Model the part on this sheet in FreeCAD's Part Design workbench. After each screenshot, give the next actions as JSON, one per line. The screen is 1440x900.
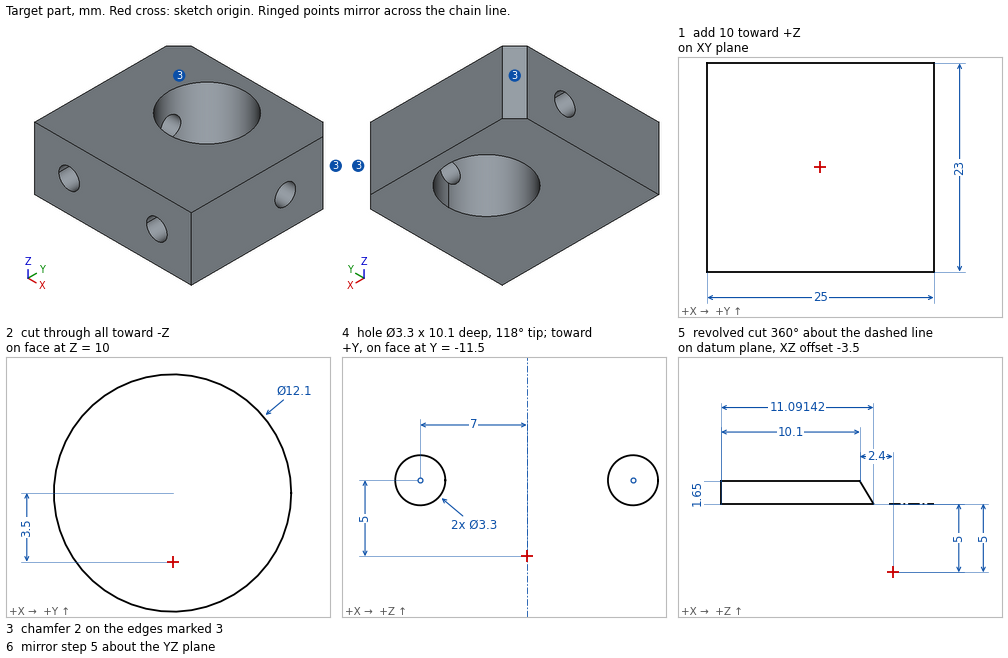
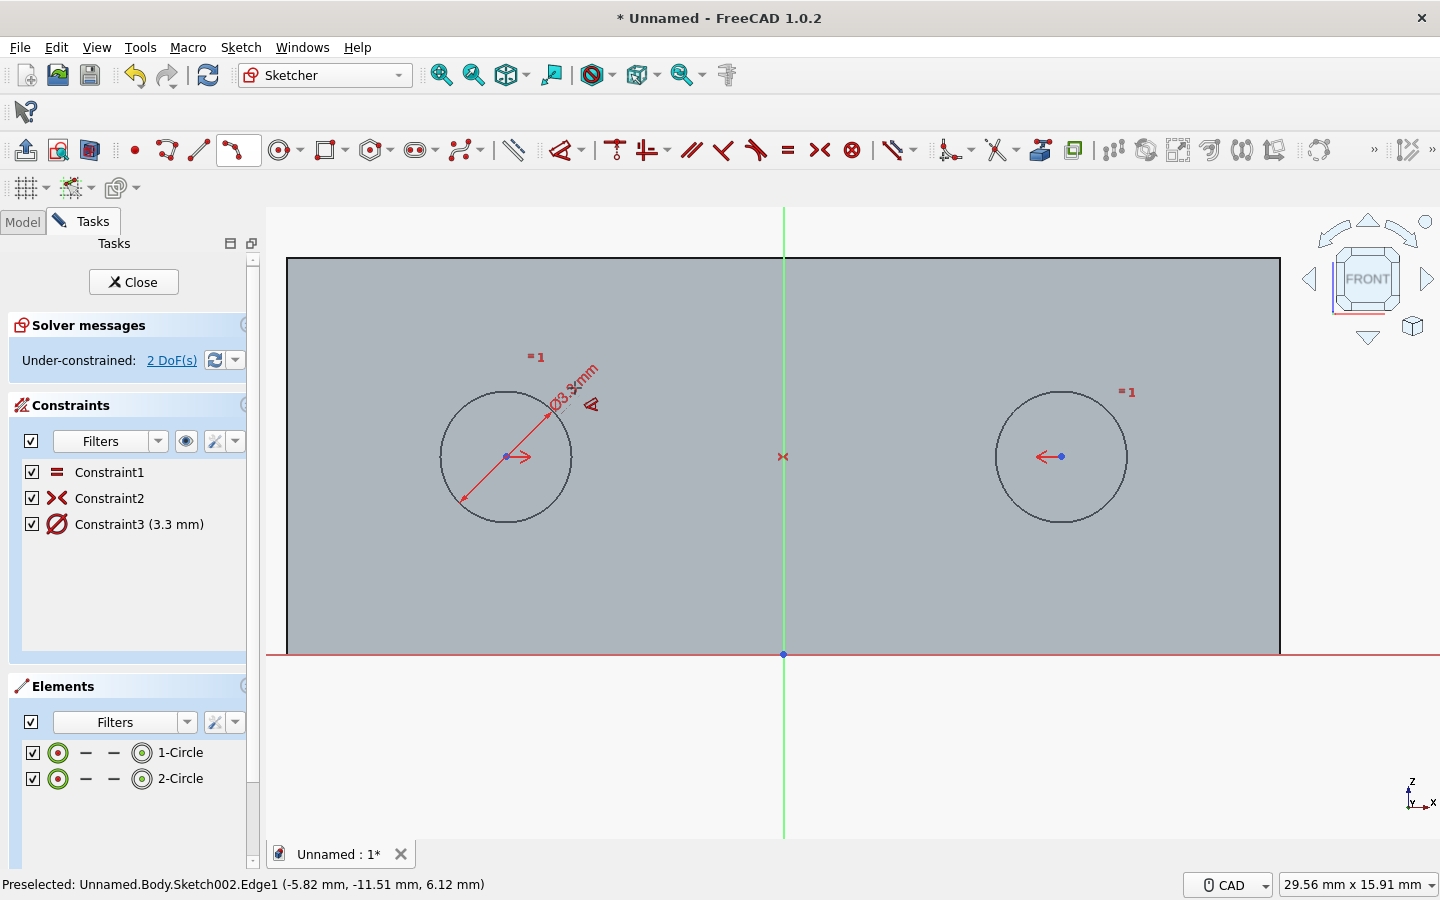
{"action": "left_click", "coordinate": [506, 457]}
{"action": "left_click", "coordinate": [645, 689]}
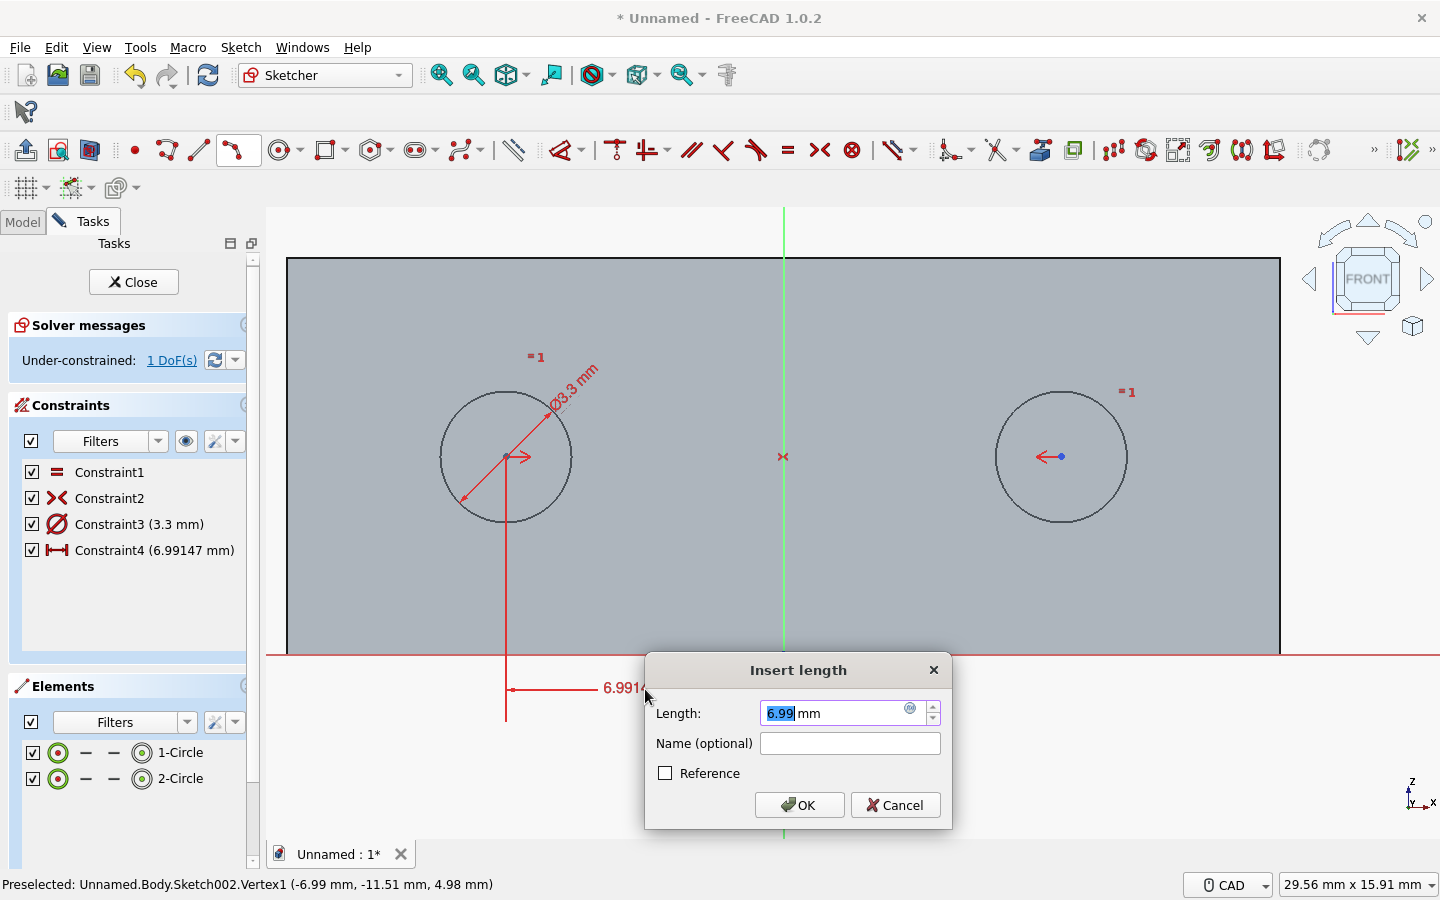
{"action": "type", "text": "7"}
{"action": "key", "text": "Return"}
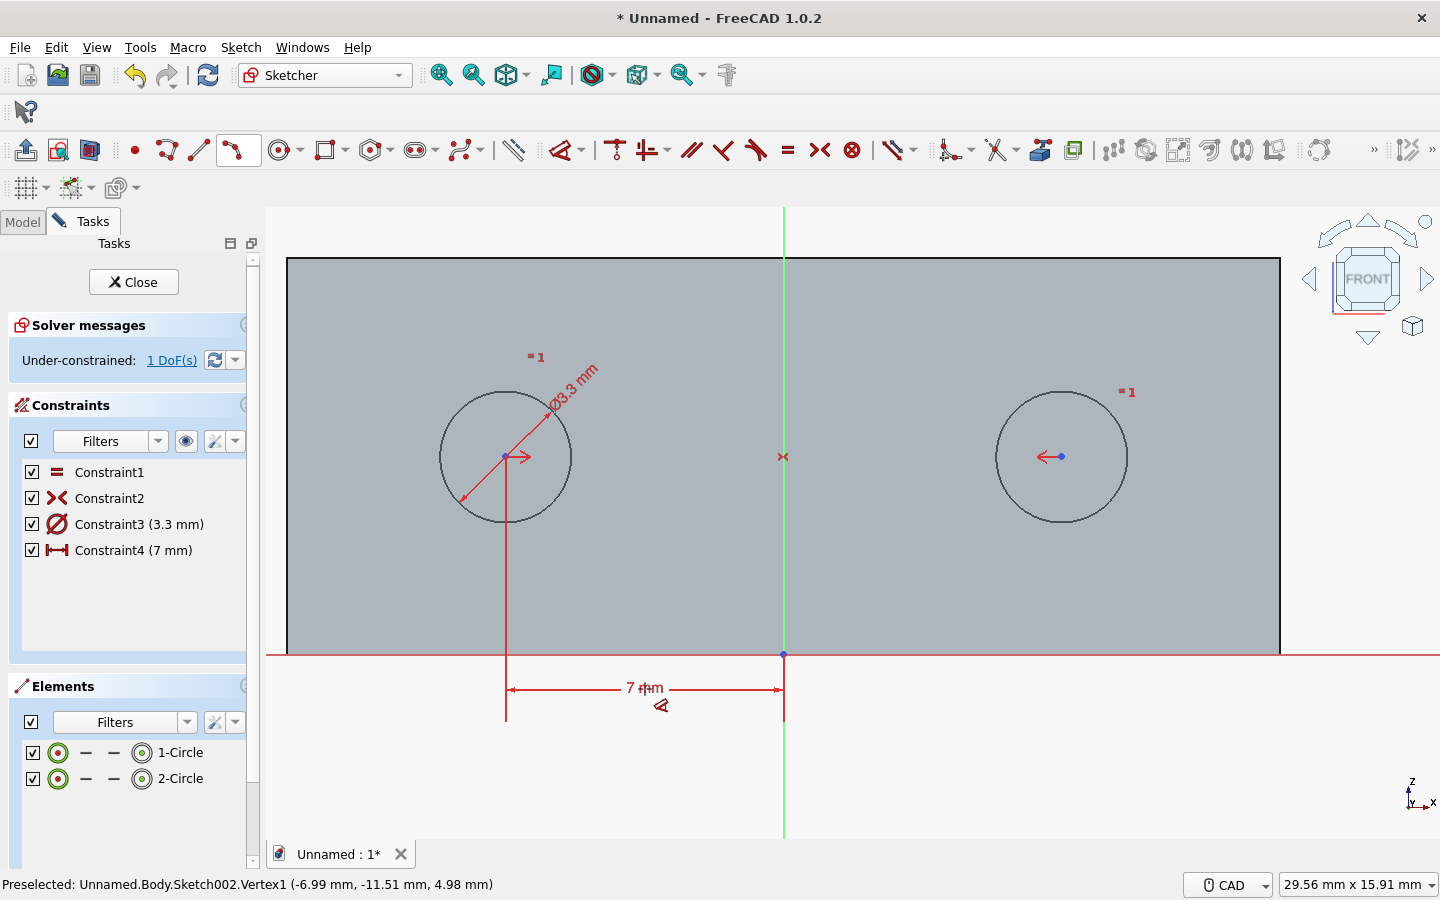
{"action": "left_click", "coordinate": [506, 457]}
{"action": "left_click", "coordinate": [472, 556]}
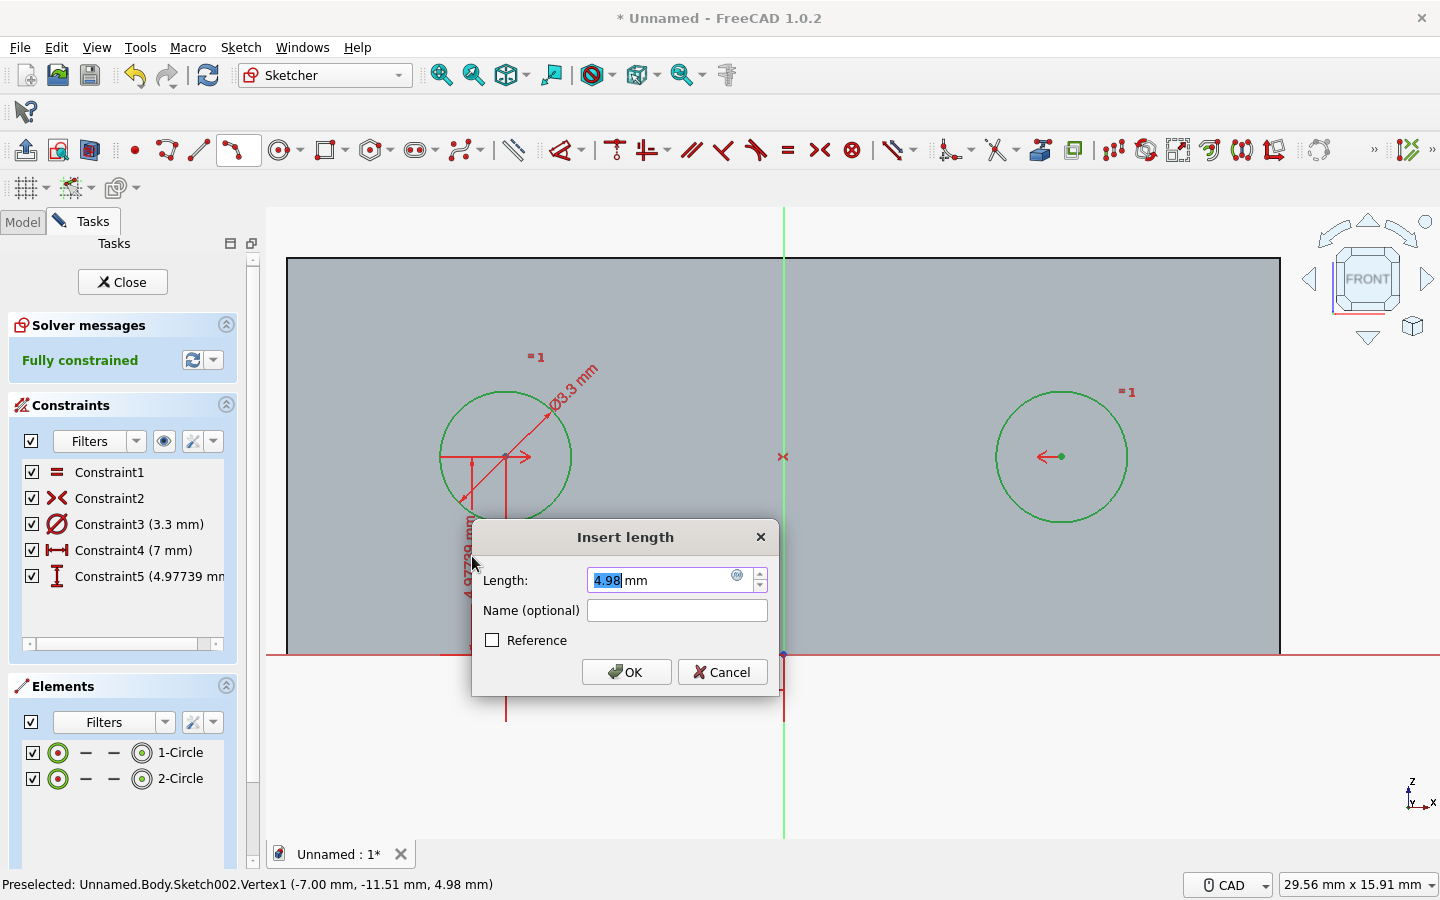
{"action": "type", "text": "5"}
{"action": "key", "text": "Return"}
{"action": "key", "text": "Escape"}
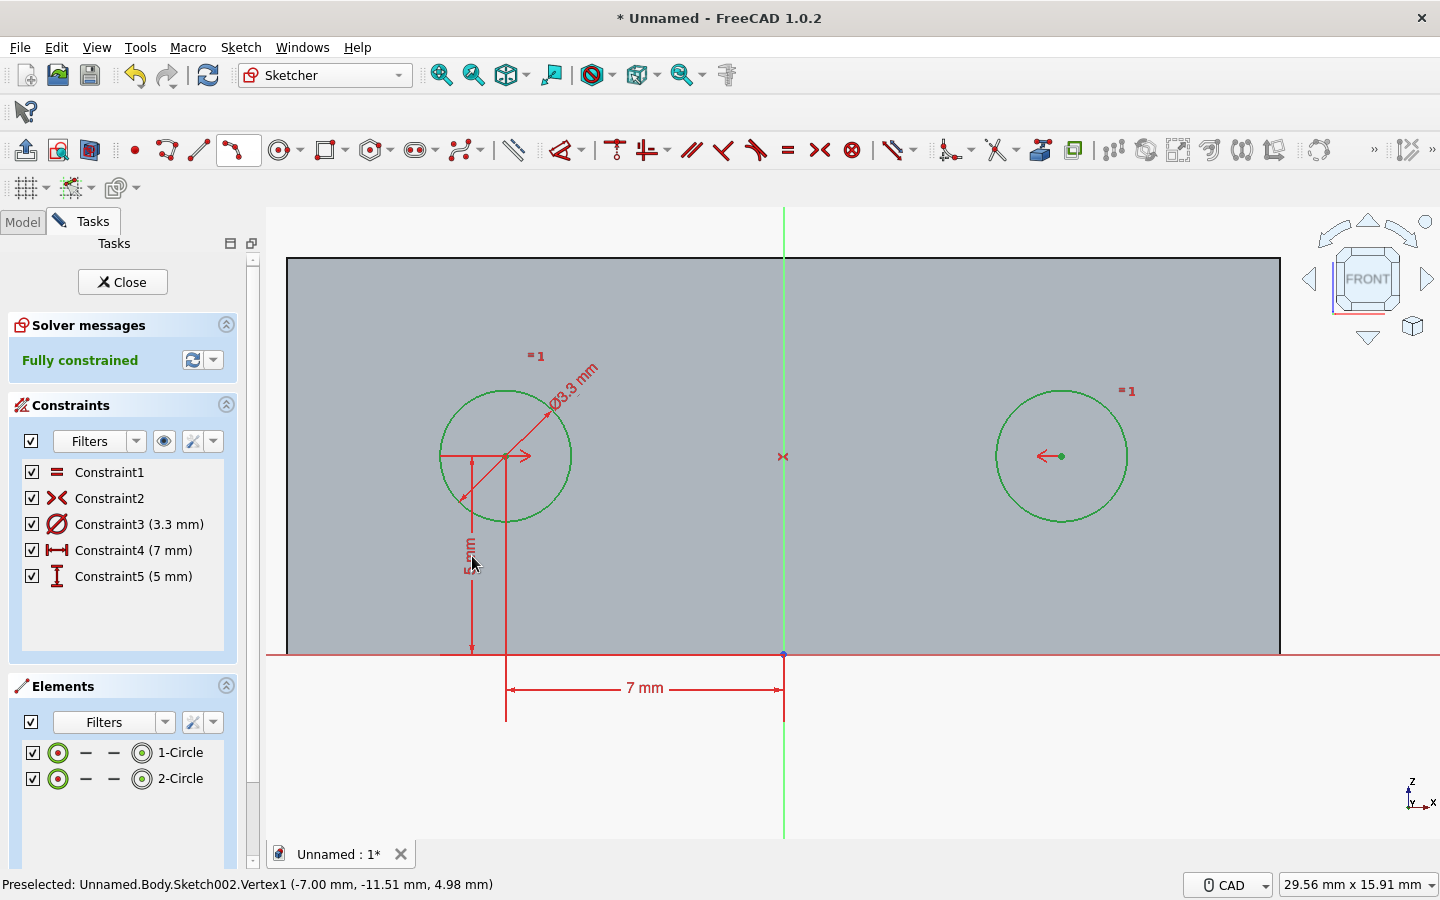
{"action": "left_click", "coordinate": [123, 282]}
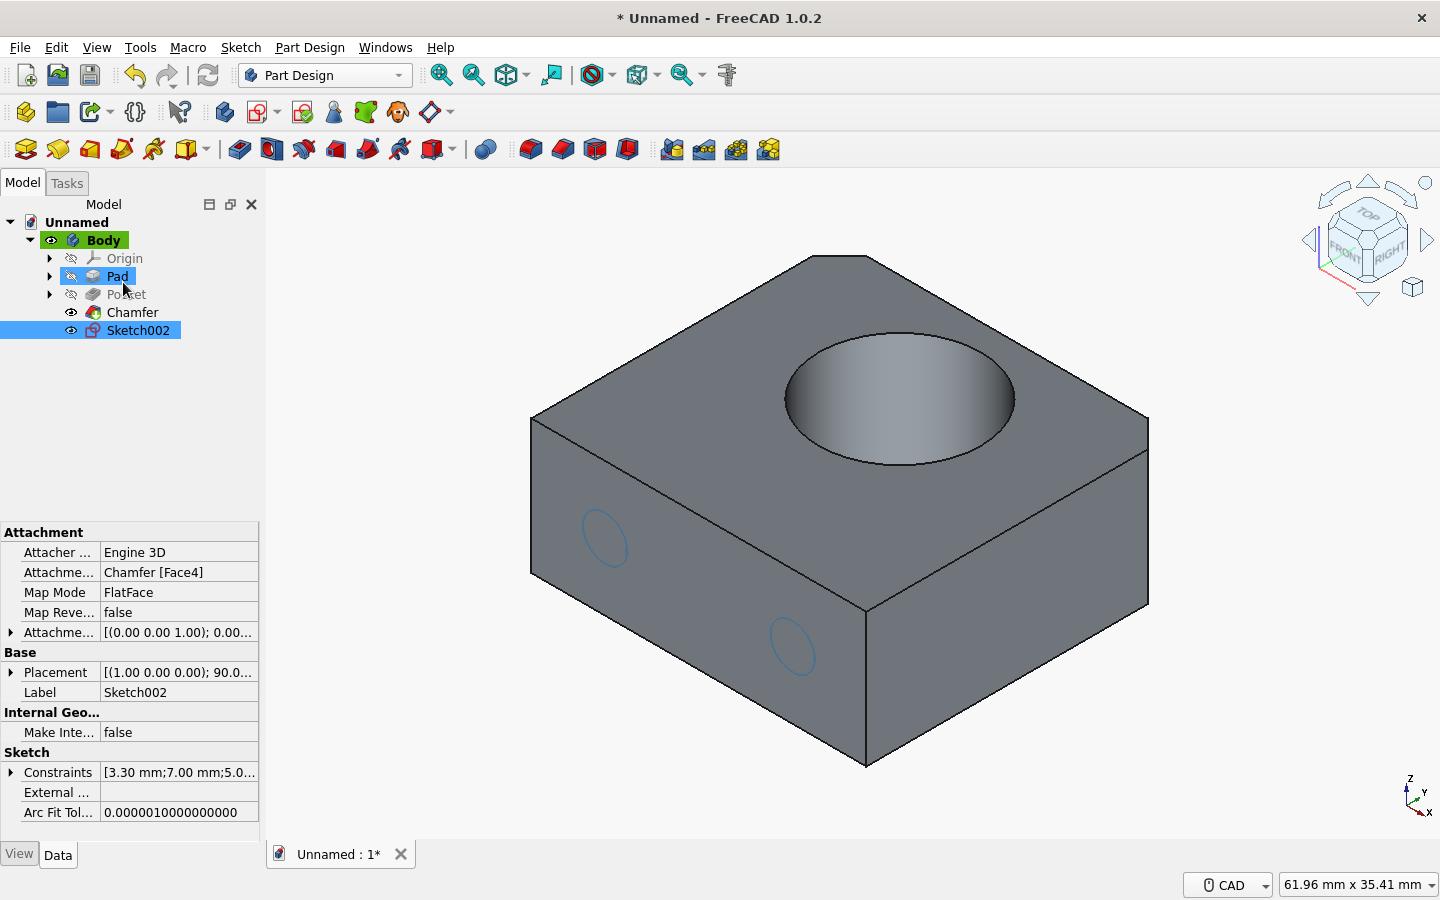
{"action": "left_click", "coordinate": [272, 150]}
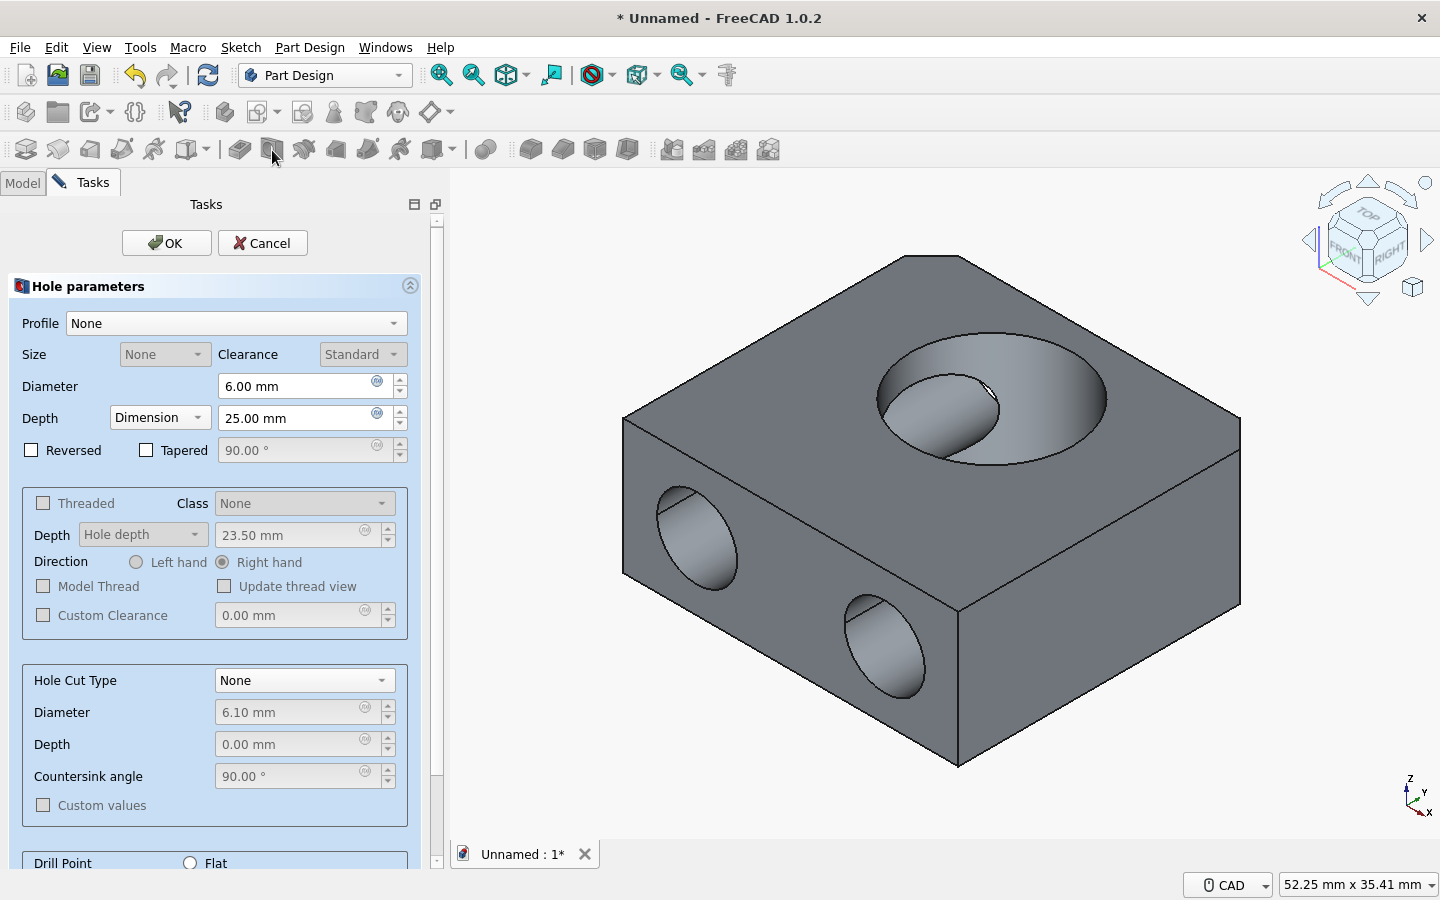
{"action": "triple_click", "coordinate": [305, 386]}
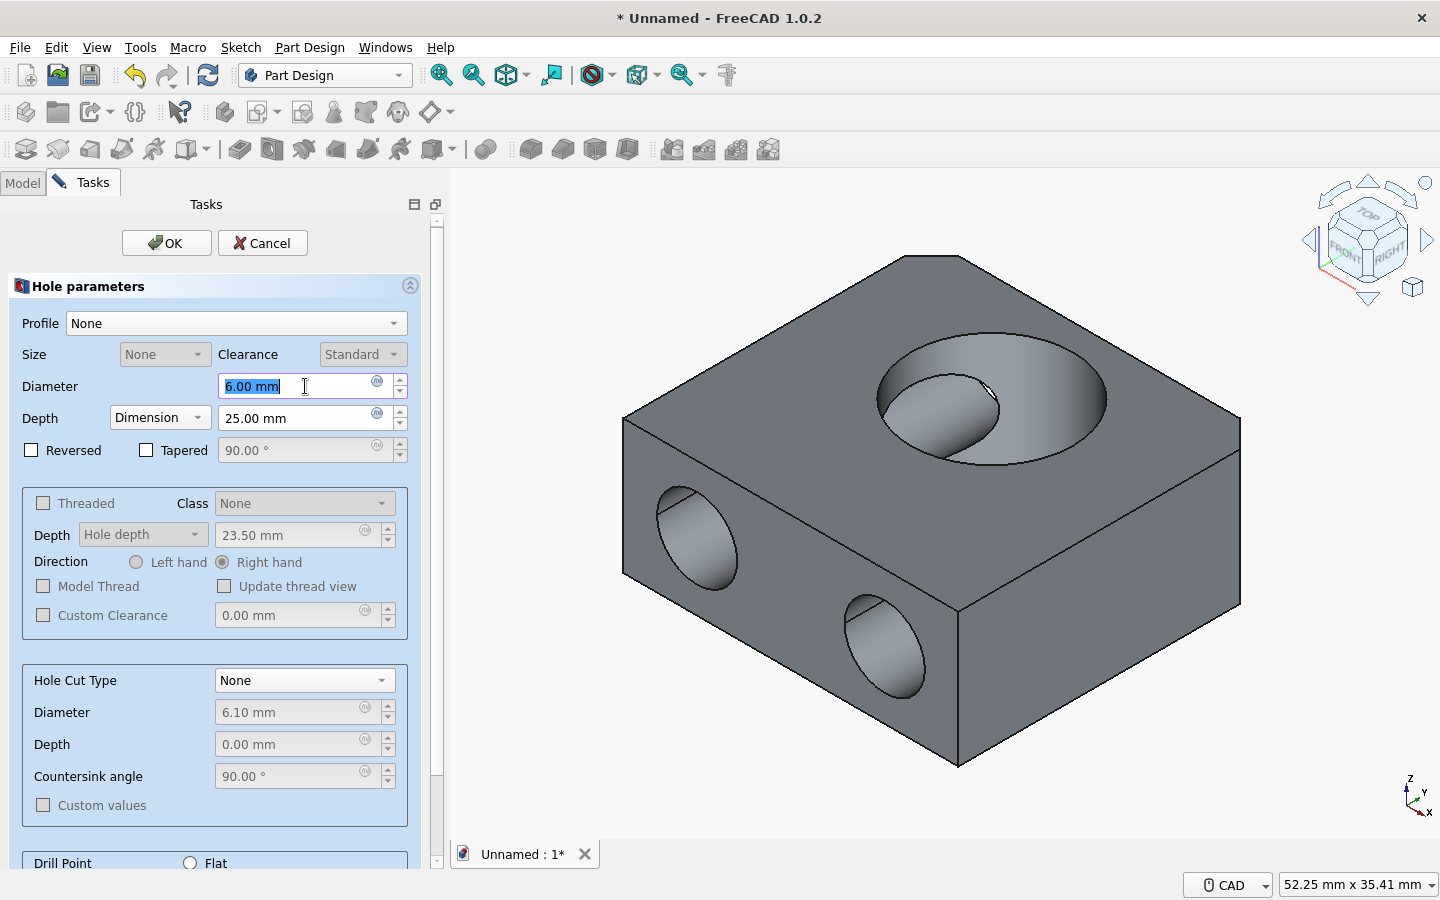
{"action": "type", "text": "3.3"}
{"action": "key", "text": "Tab"}